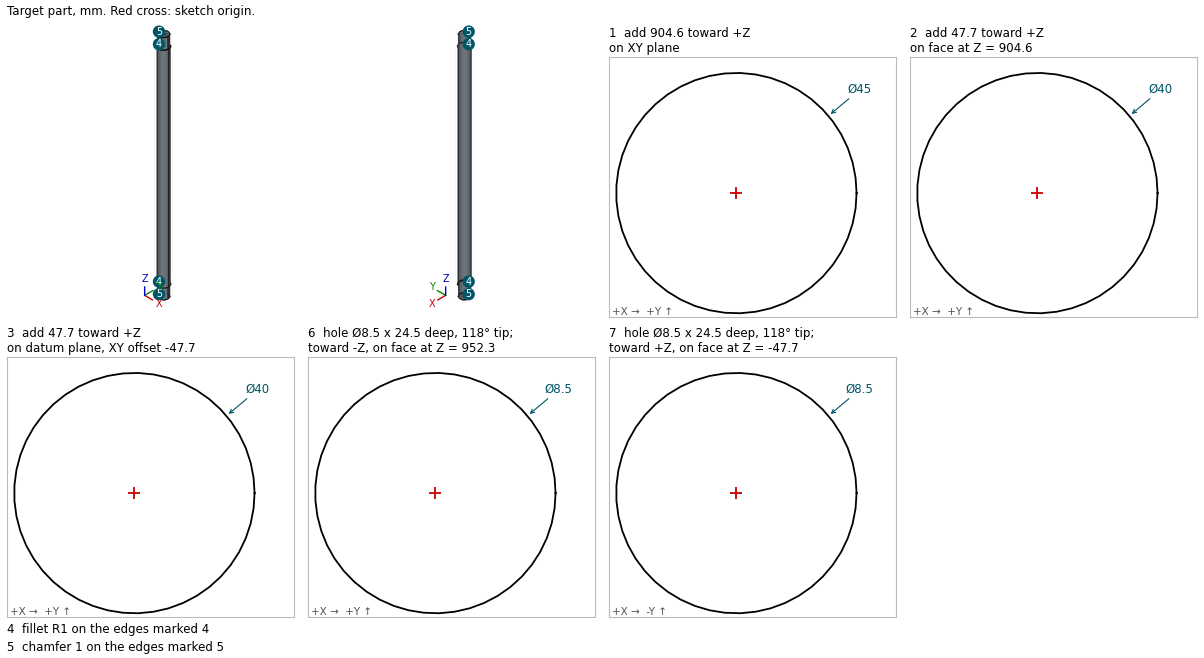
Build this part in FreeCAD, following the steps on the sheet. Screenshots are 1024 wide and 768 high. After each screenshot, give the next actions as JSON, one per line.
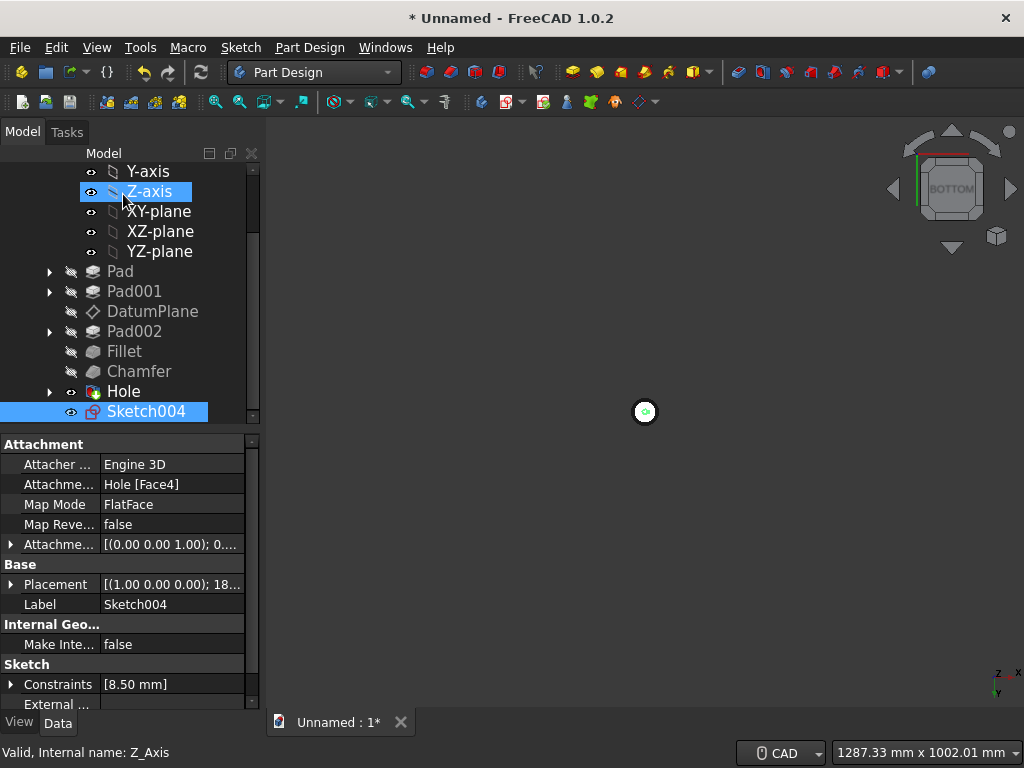
{"action": "left_click", "coordinate": [764, 72]}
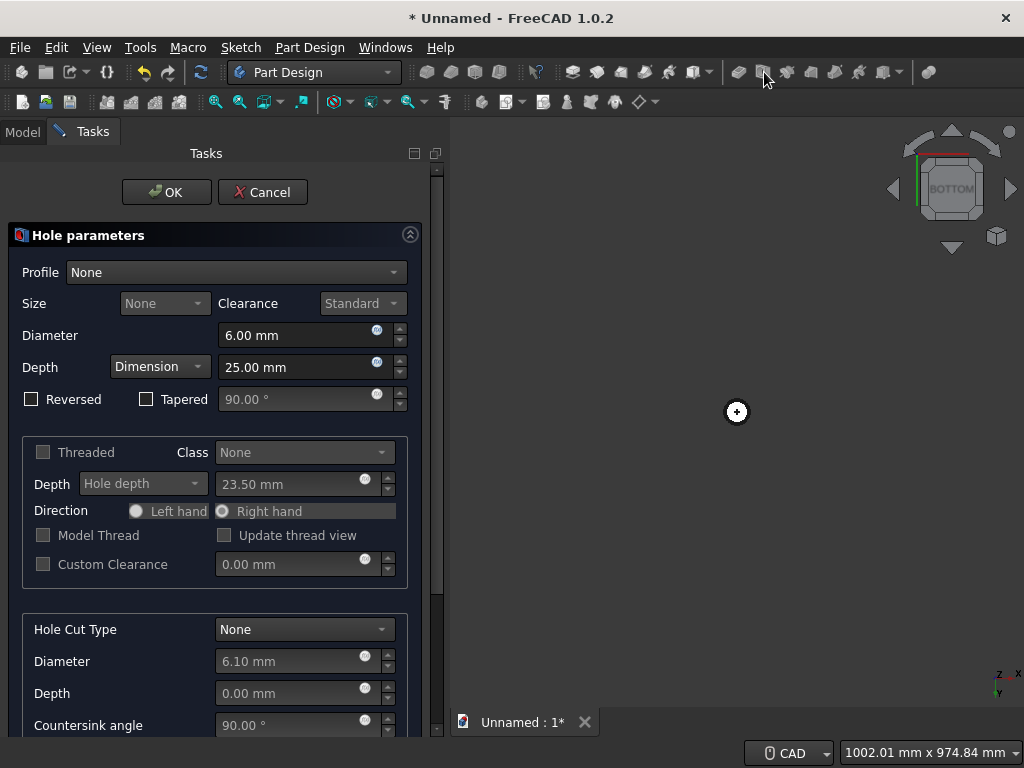
{"action": "triple_click", "coordinate": [305, 335]}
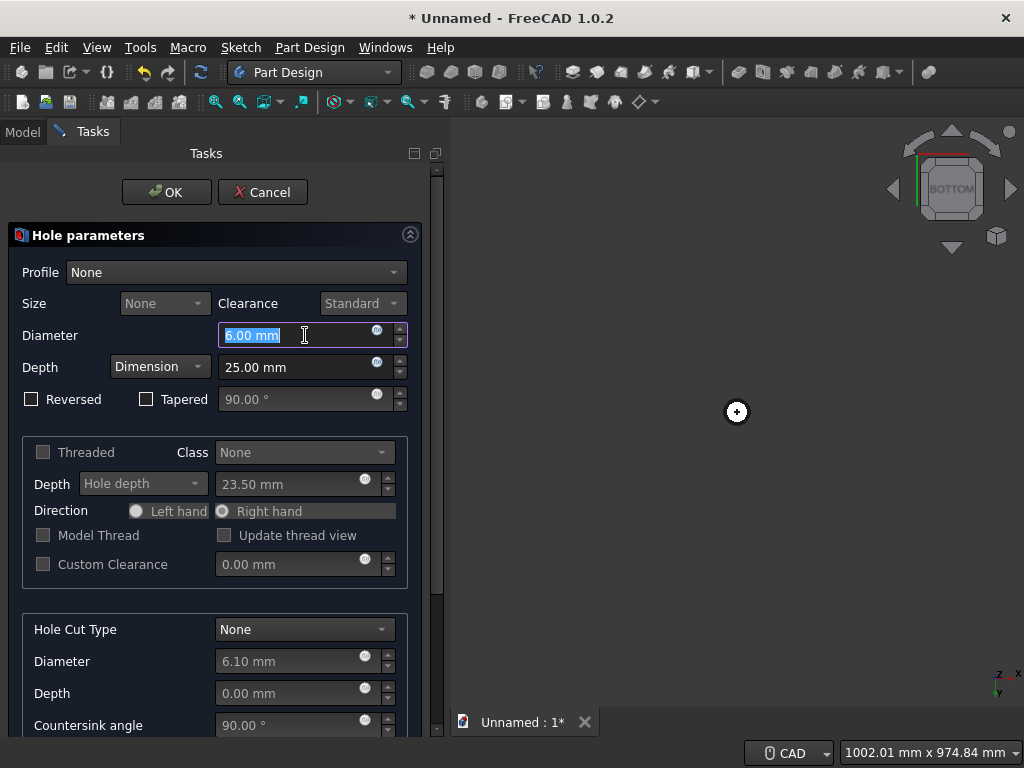
{"action": "type", "text": "8.5"}
{"action": "key", "text": "Tab"}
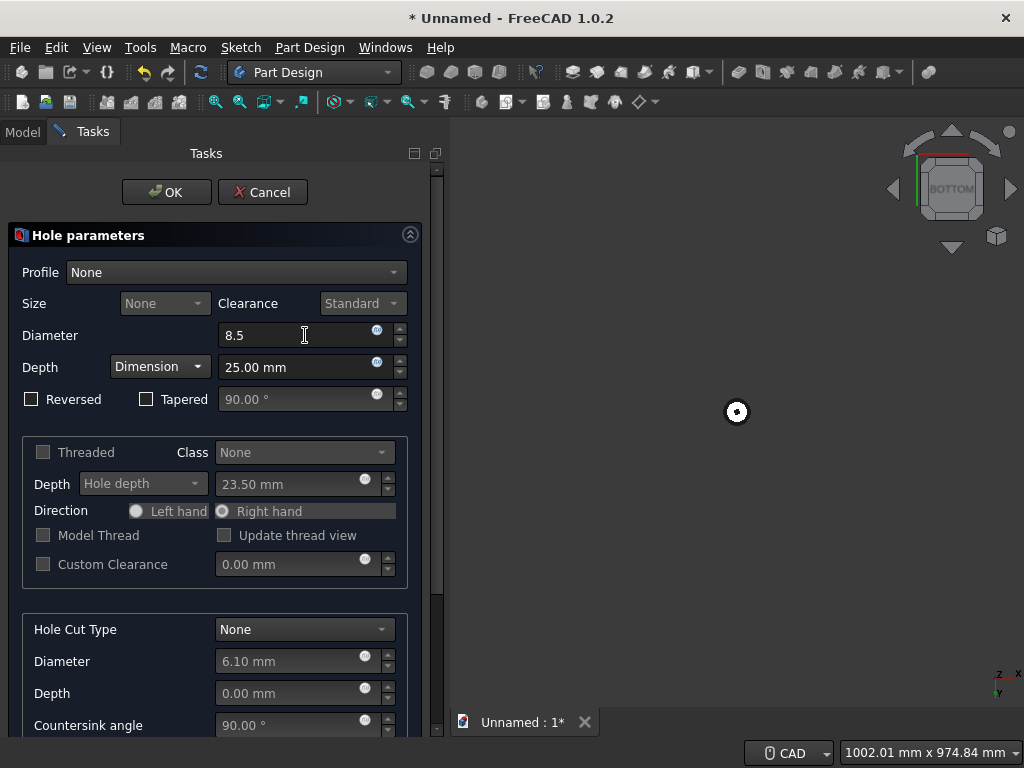
{"action": "triple_click", "coordinate": [305, 367]}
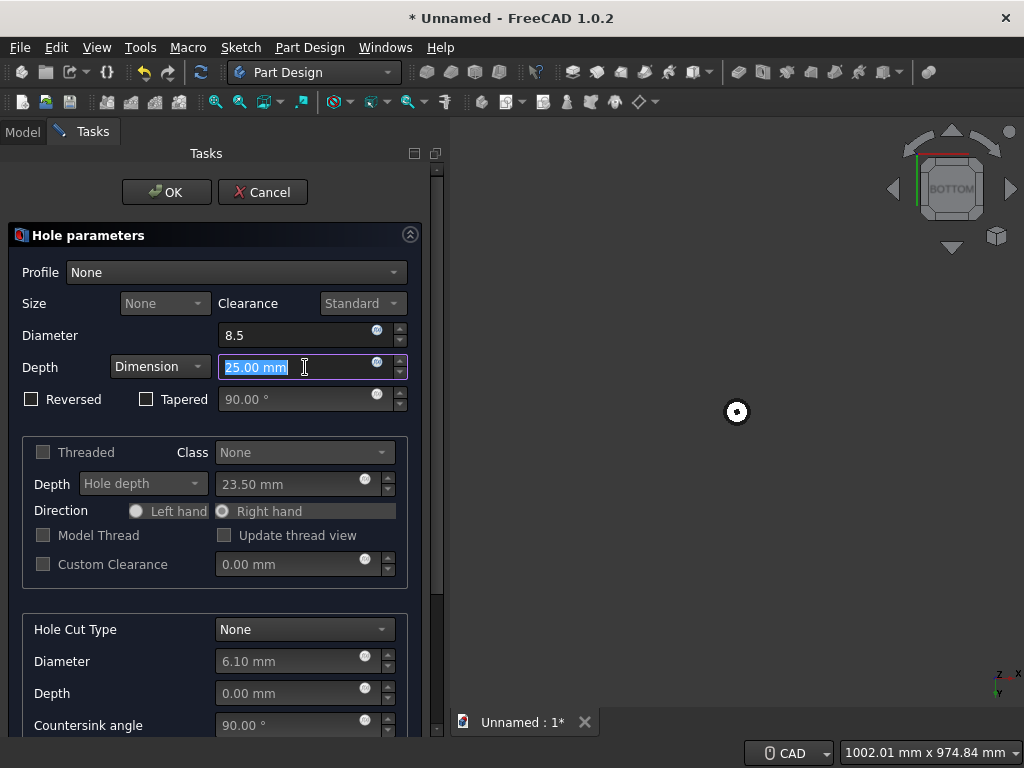
{"action": "type", "text": "24.5"}
{"action": "key", "text": "Tab"}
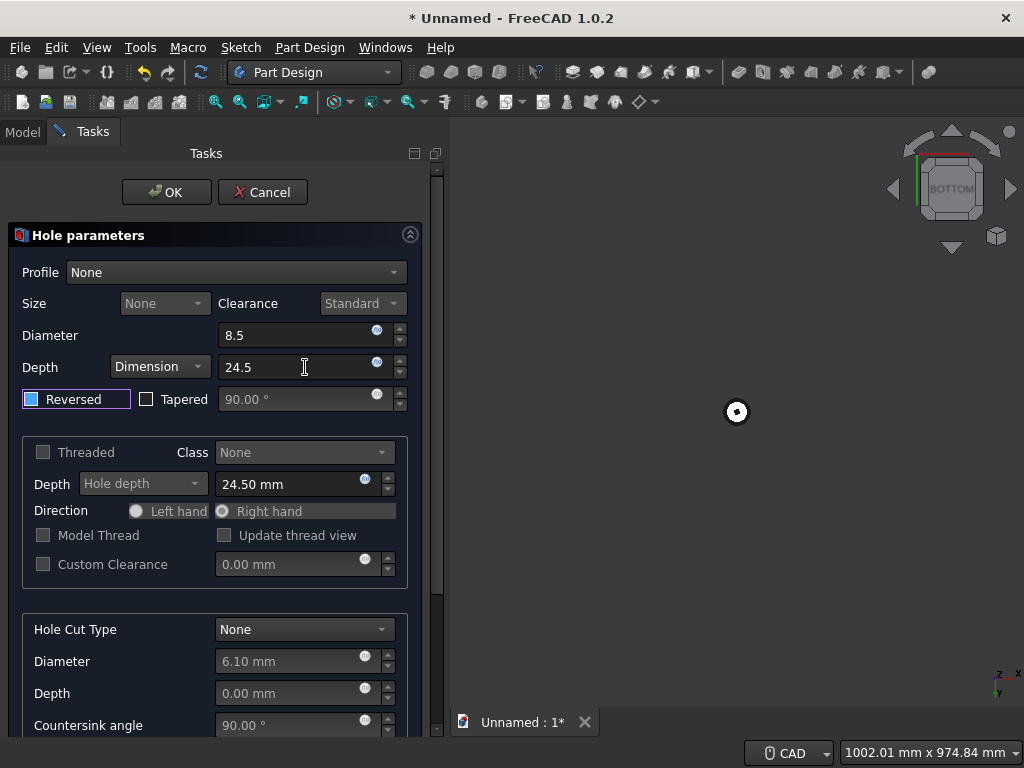
{"action": "left_click", "coordinate": [167, 192]}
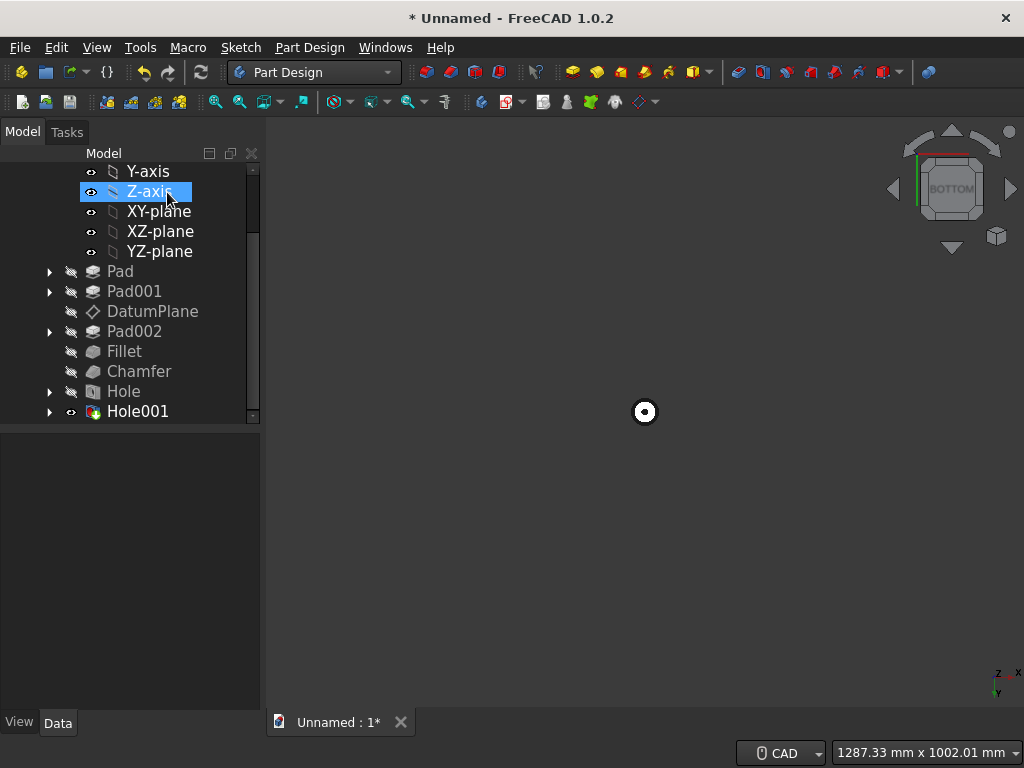
{"action": "key", "text": "0"}